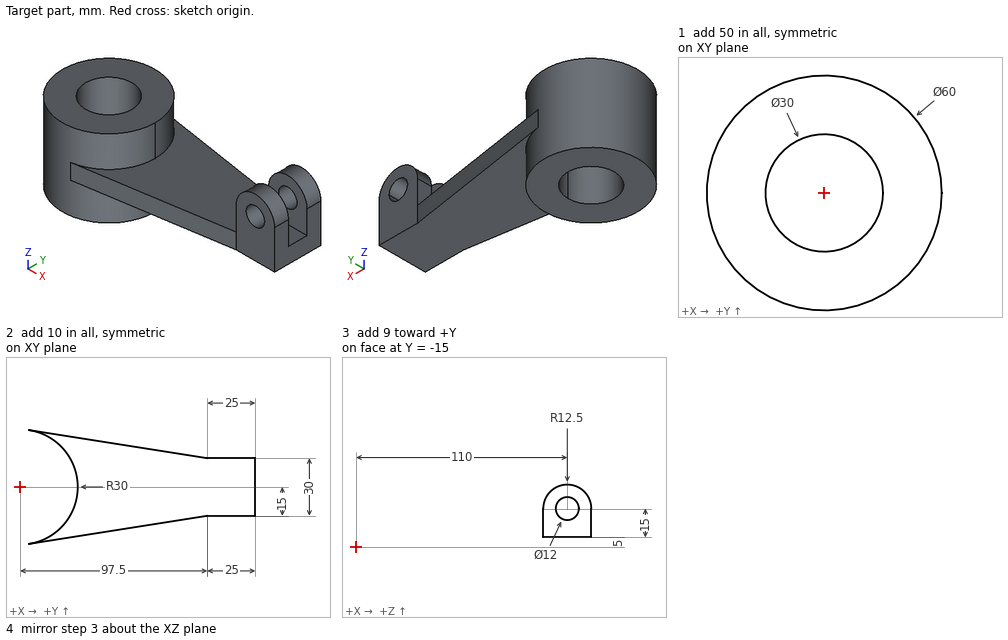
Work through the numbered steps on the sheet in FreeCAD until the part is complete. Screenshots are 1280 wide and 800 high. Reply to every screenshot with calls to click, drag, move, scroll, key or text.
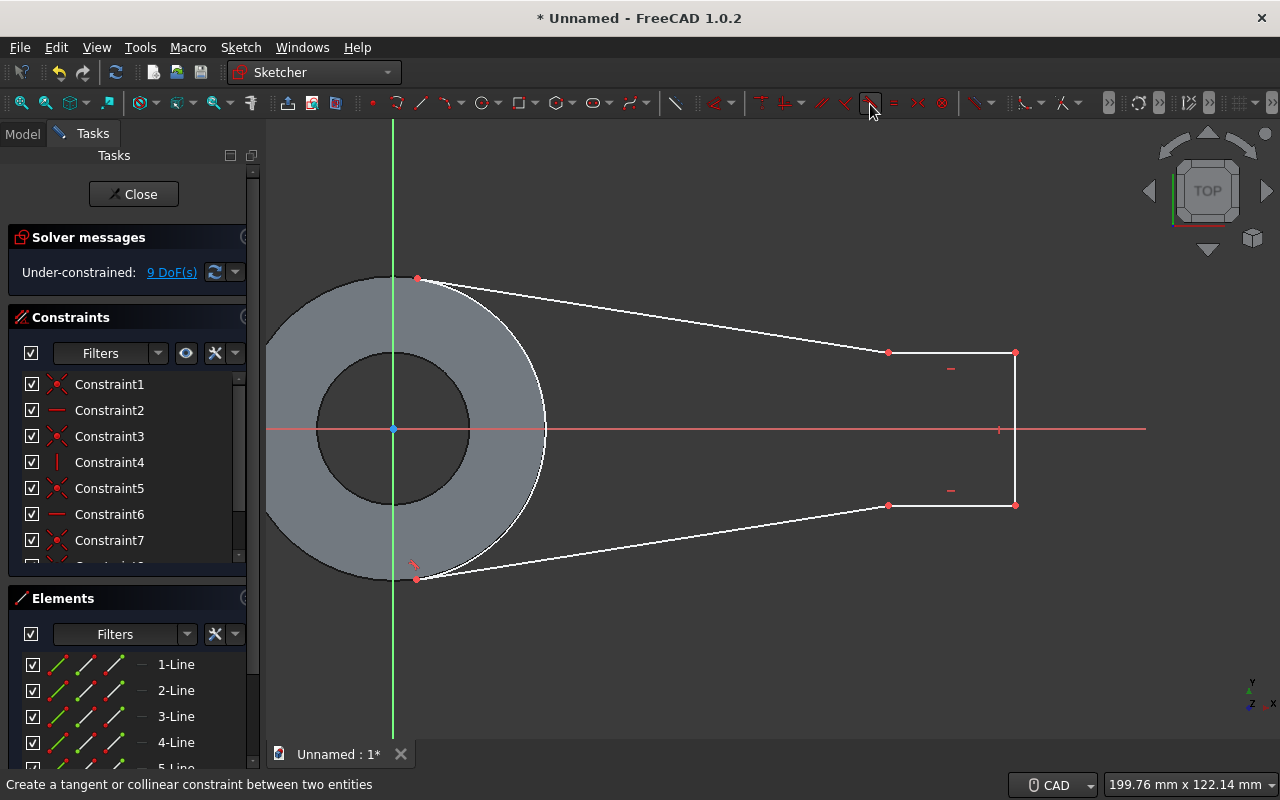
click(747, 331)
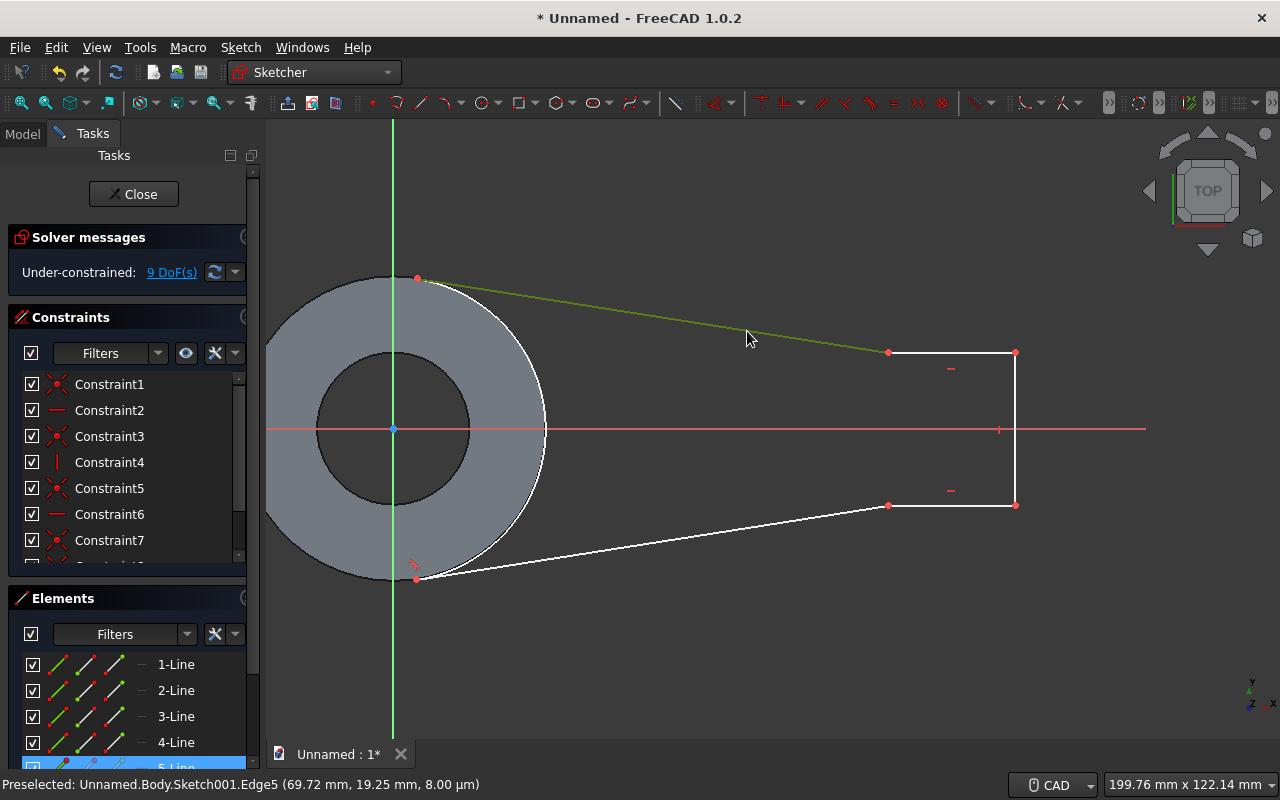
click(522, 511)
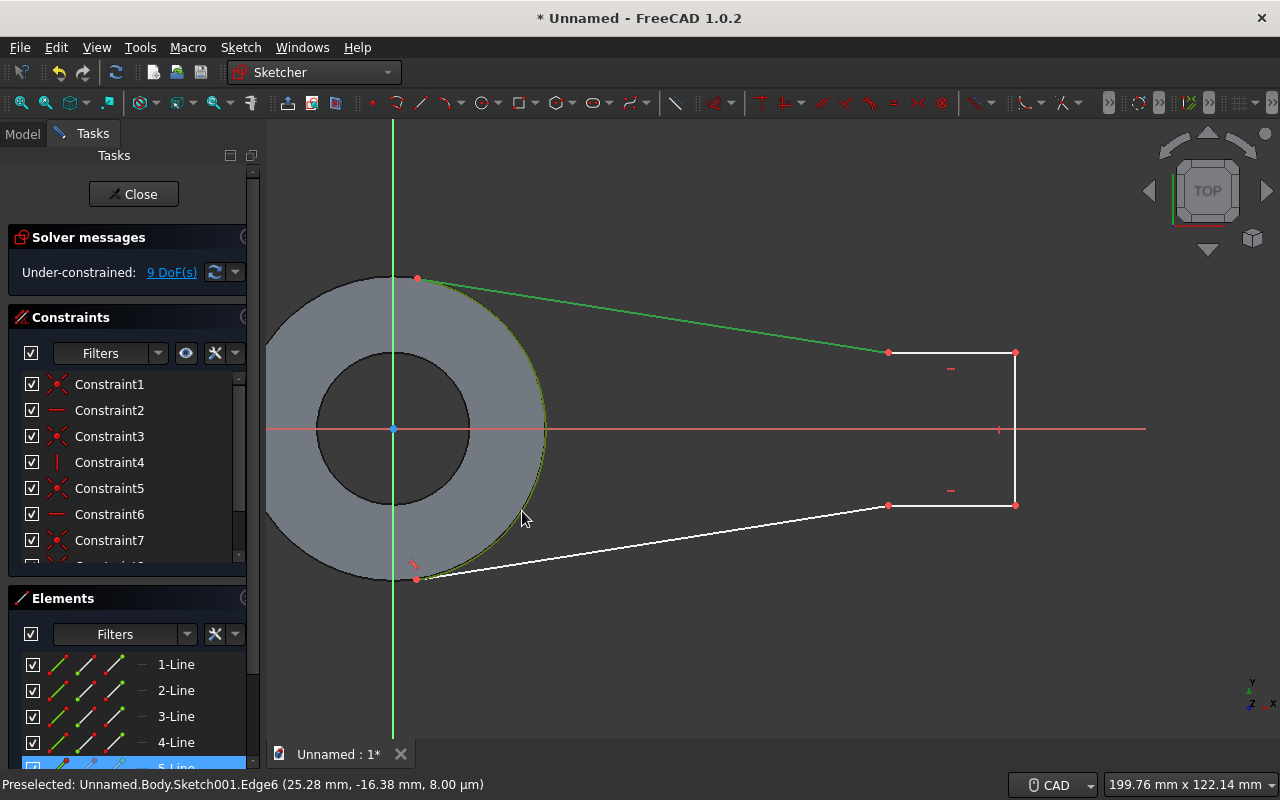
click(870, 104)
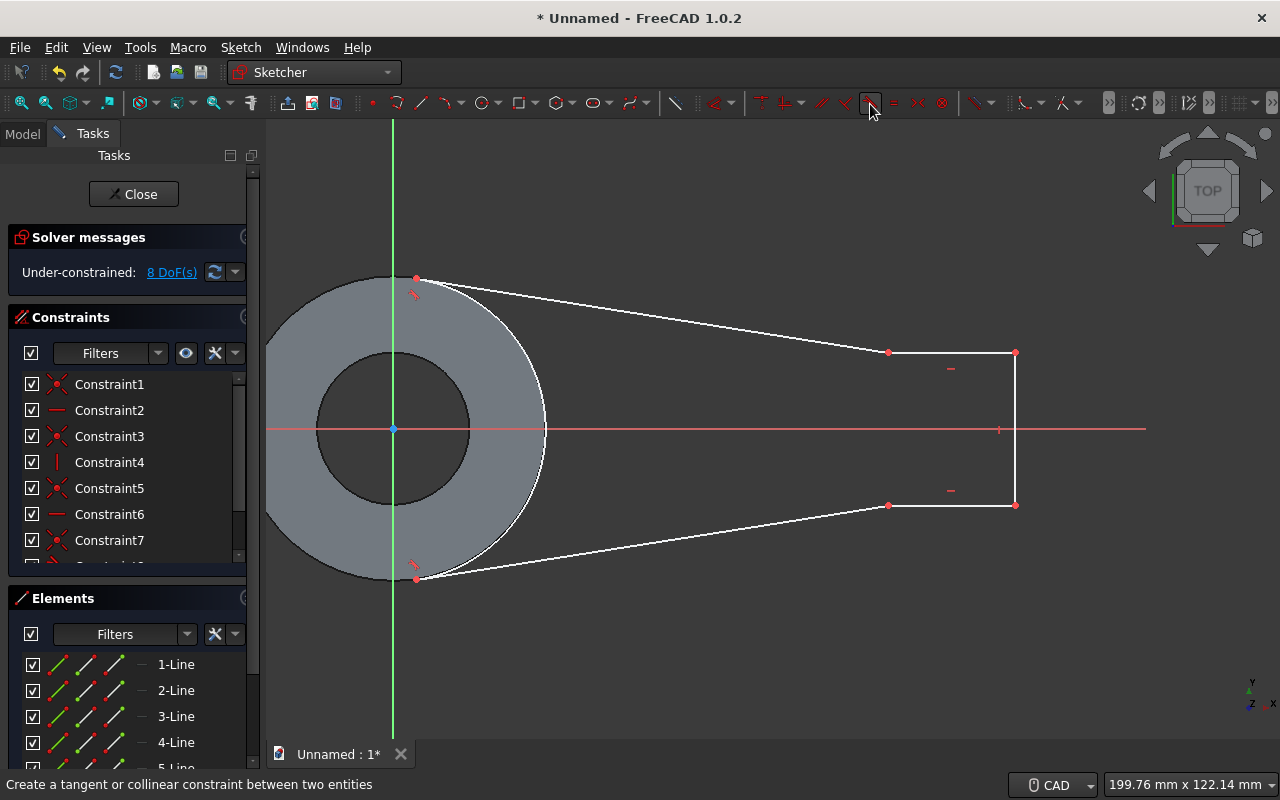
drag(383, 419, 403, 440)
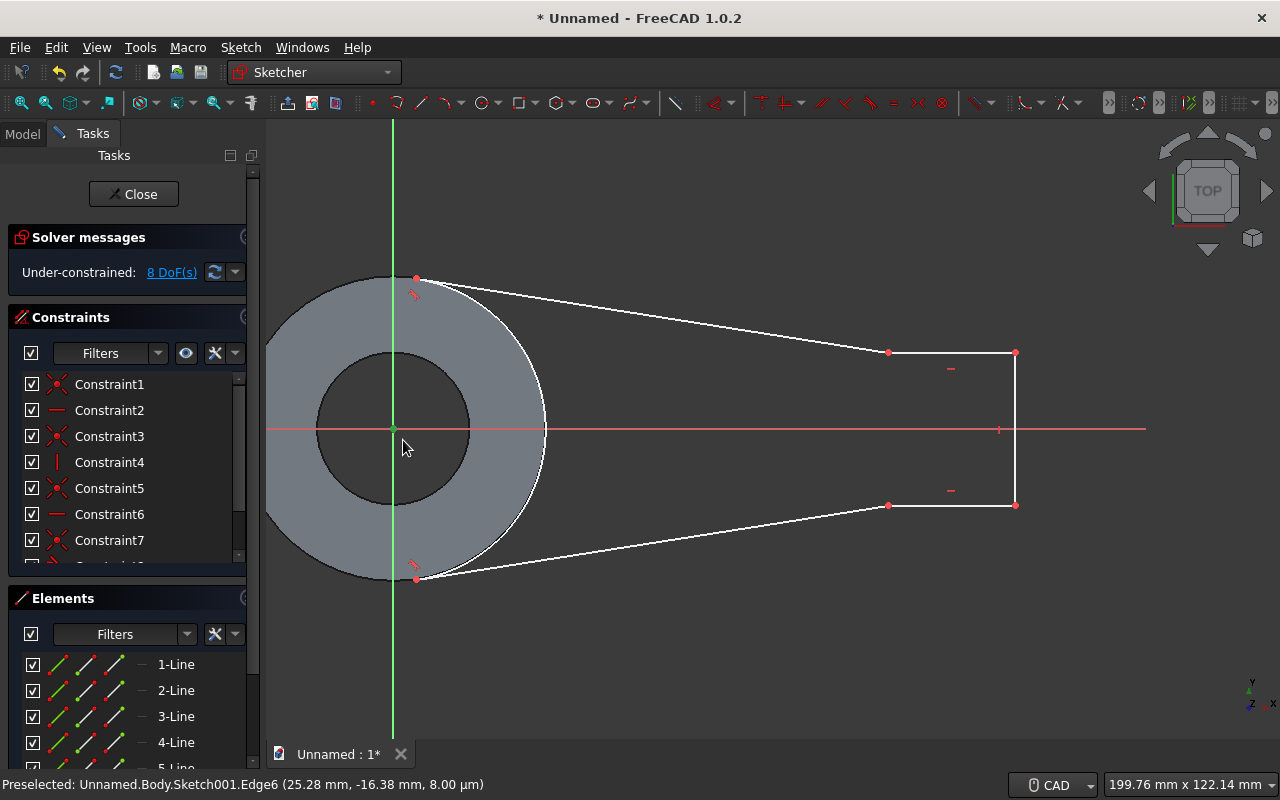
click(762, 104)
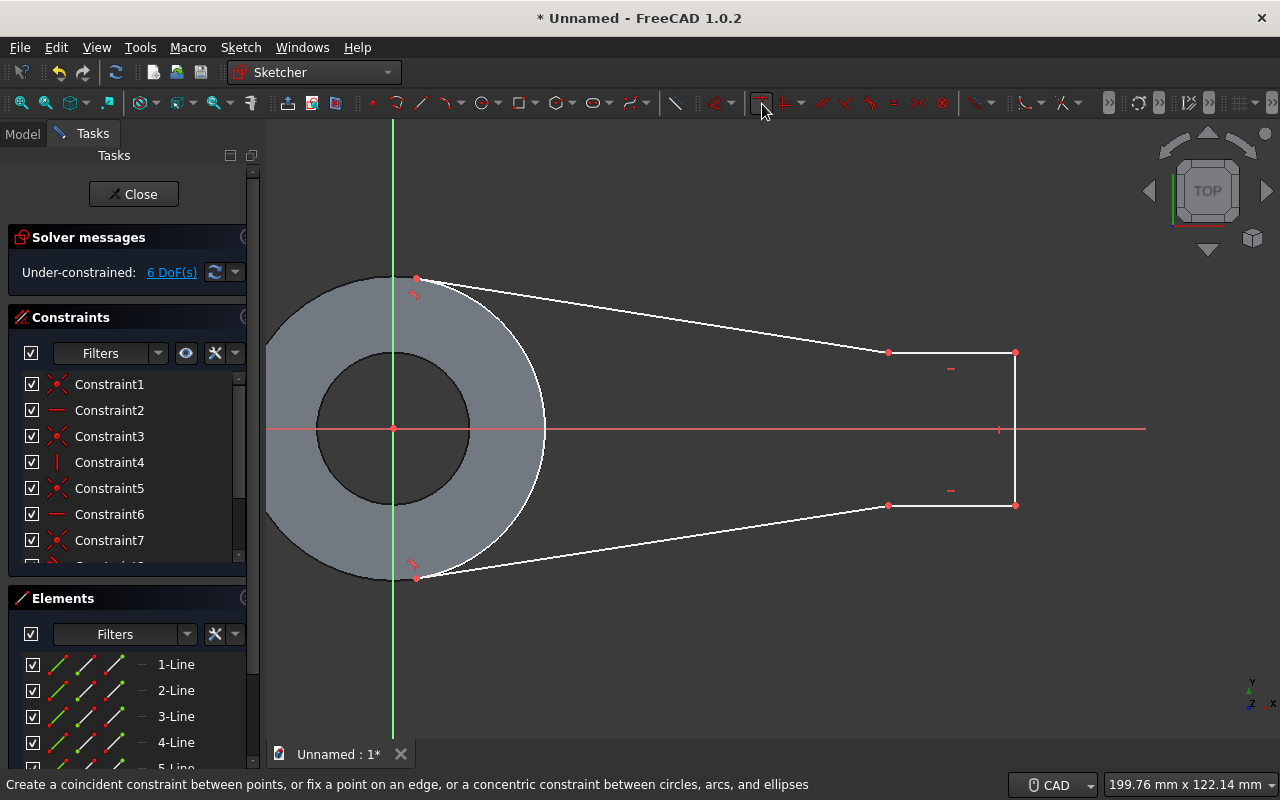
click(714, 104)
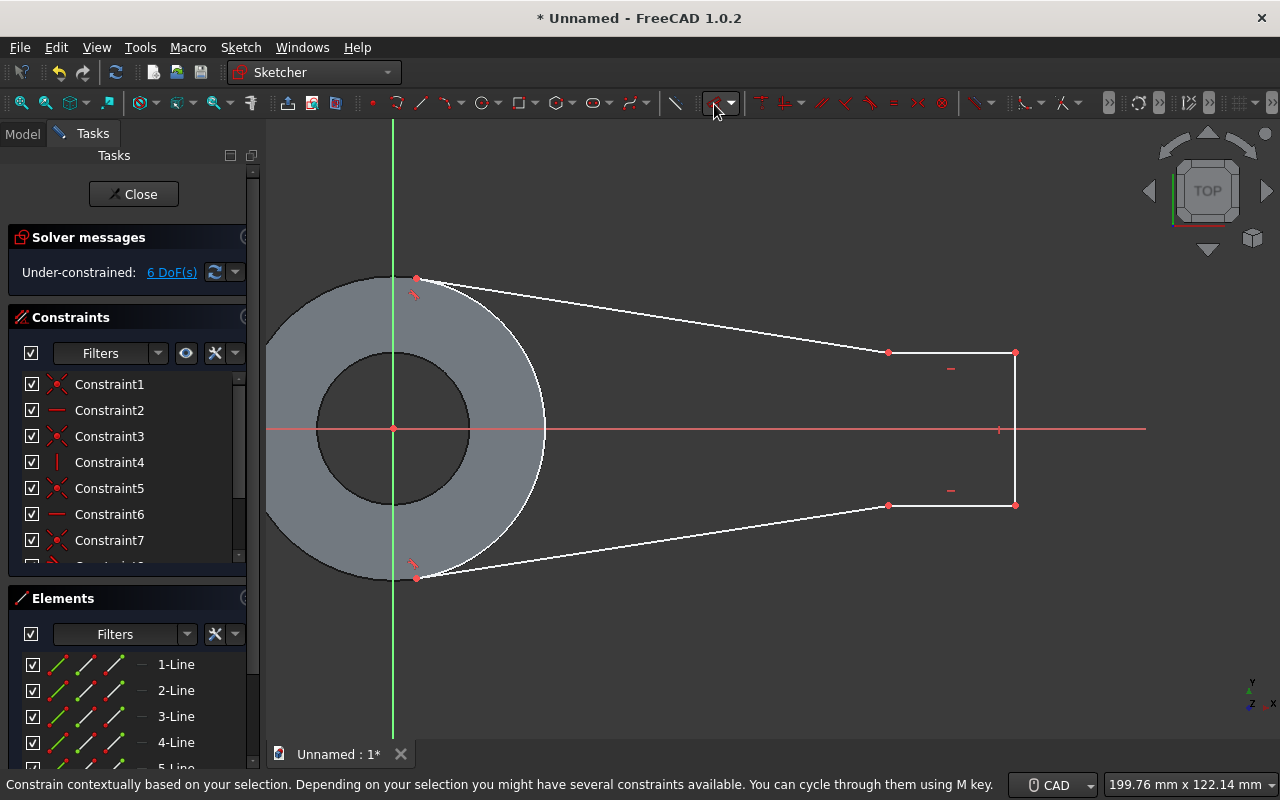
click(521, 510)
click(548, 527)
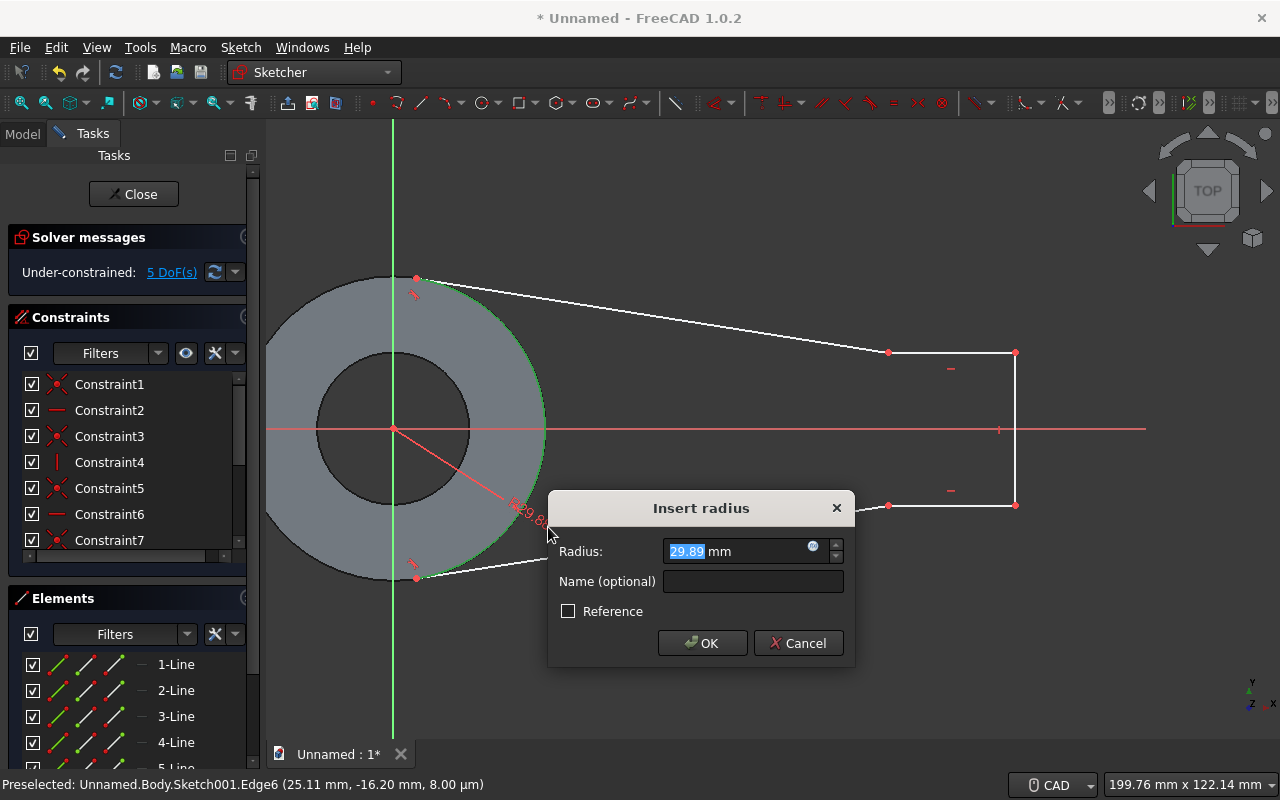
text(30)
key(Return)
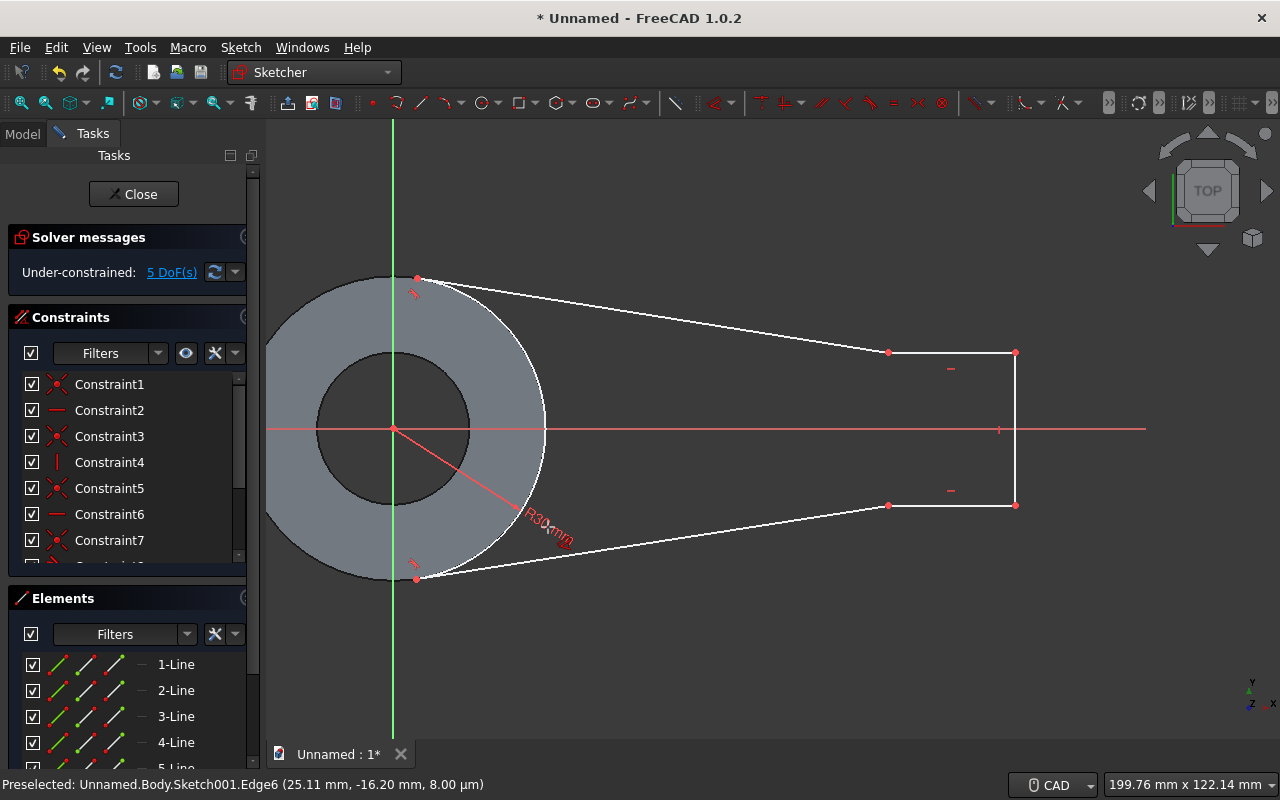
click(926, 506)
click(951, 540)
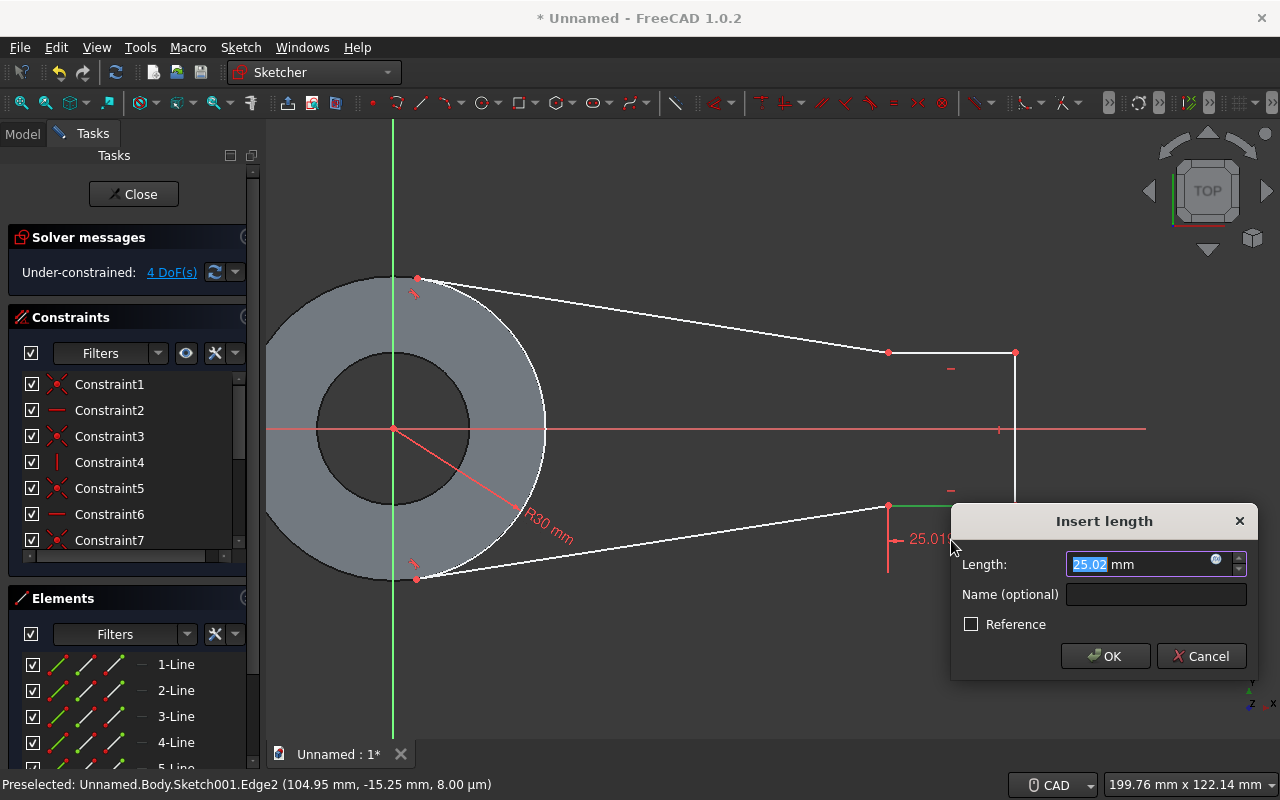
text(25)
key(Return)